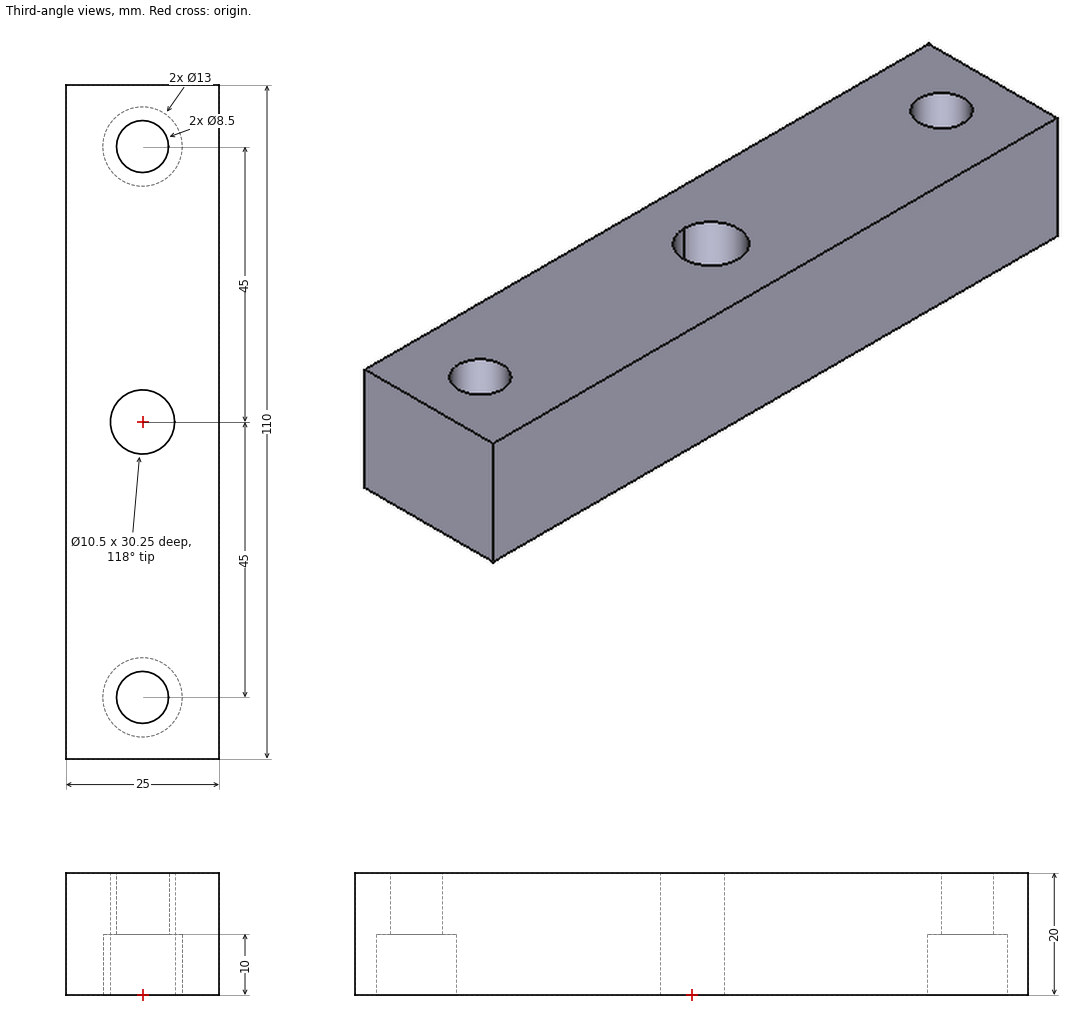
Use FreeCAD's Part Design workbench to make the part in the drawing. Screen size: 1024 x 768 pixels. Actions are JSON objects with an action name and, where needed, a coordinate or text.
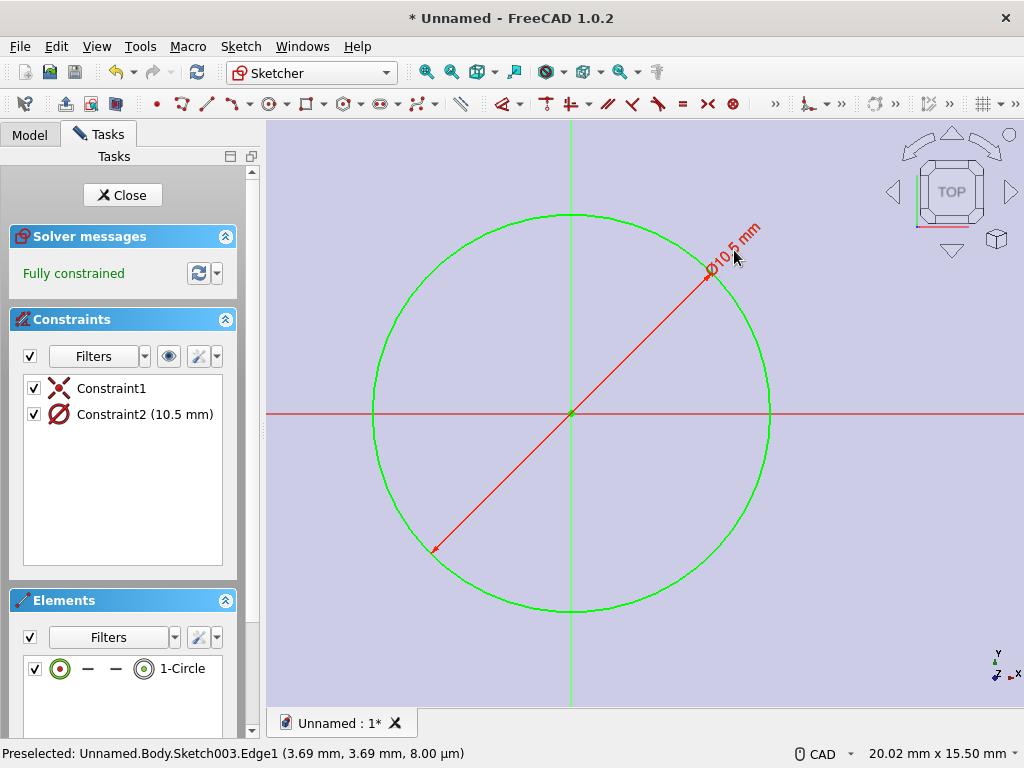
{"action": "left_click", "coordinate": [123, 195]}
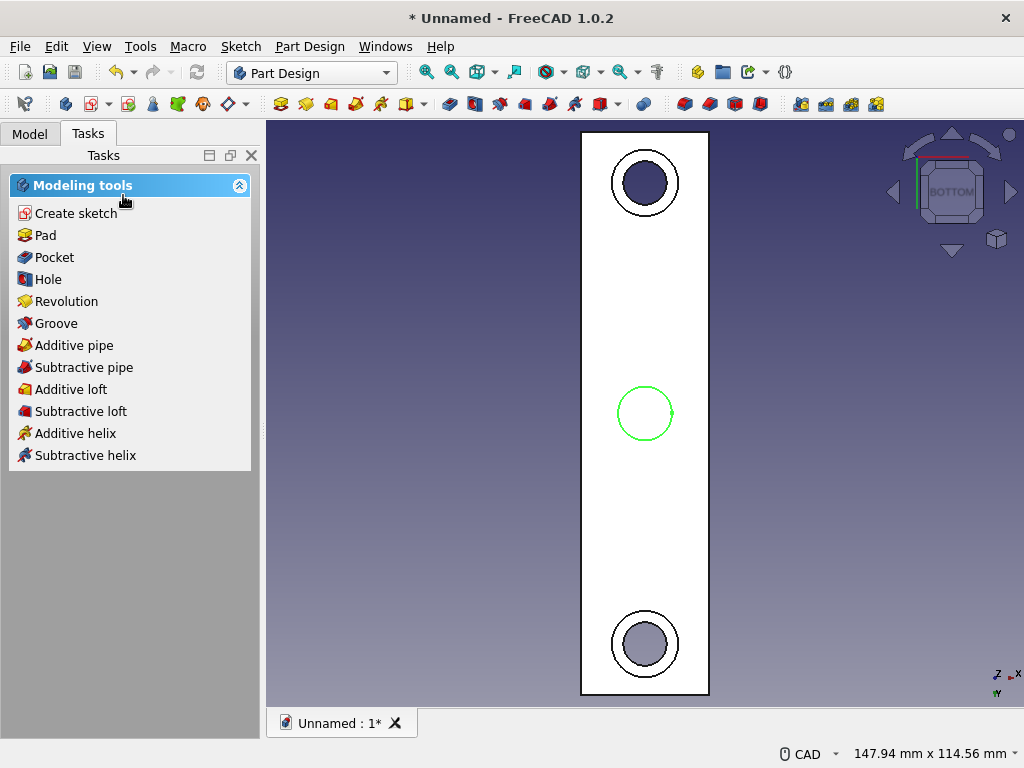
{"action": "left_click", "coordinate": [475, 104]}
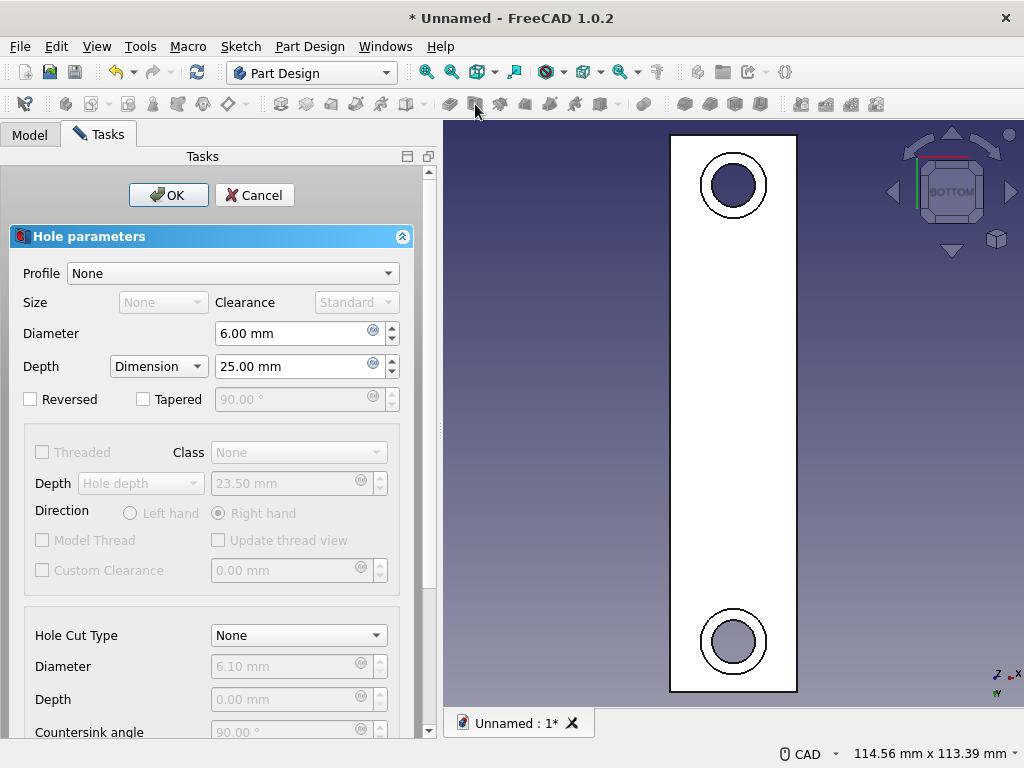
{"action": "triple_click", "coordinate": [300, 334]}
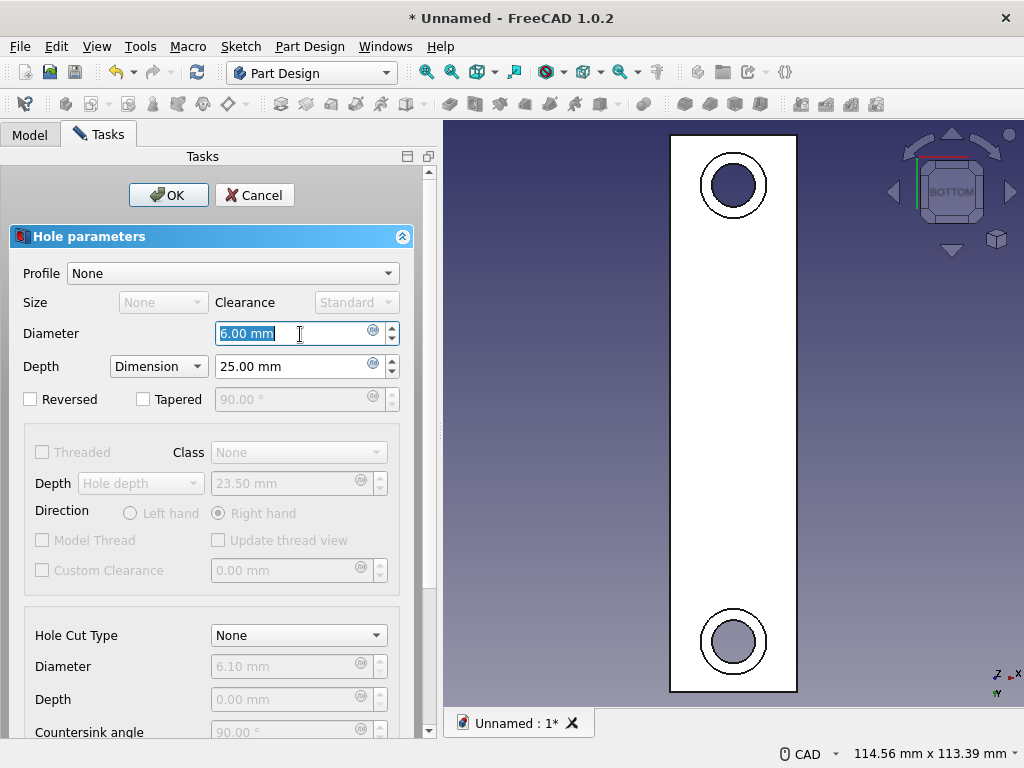
{"action": "type", "text": "10.5"}
{"action": "key", "text": "Tab"}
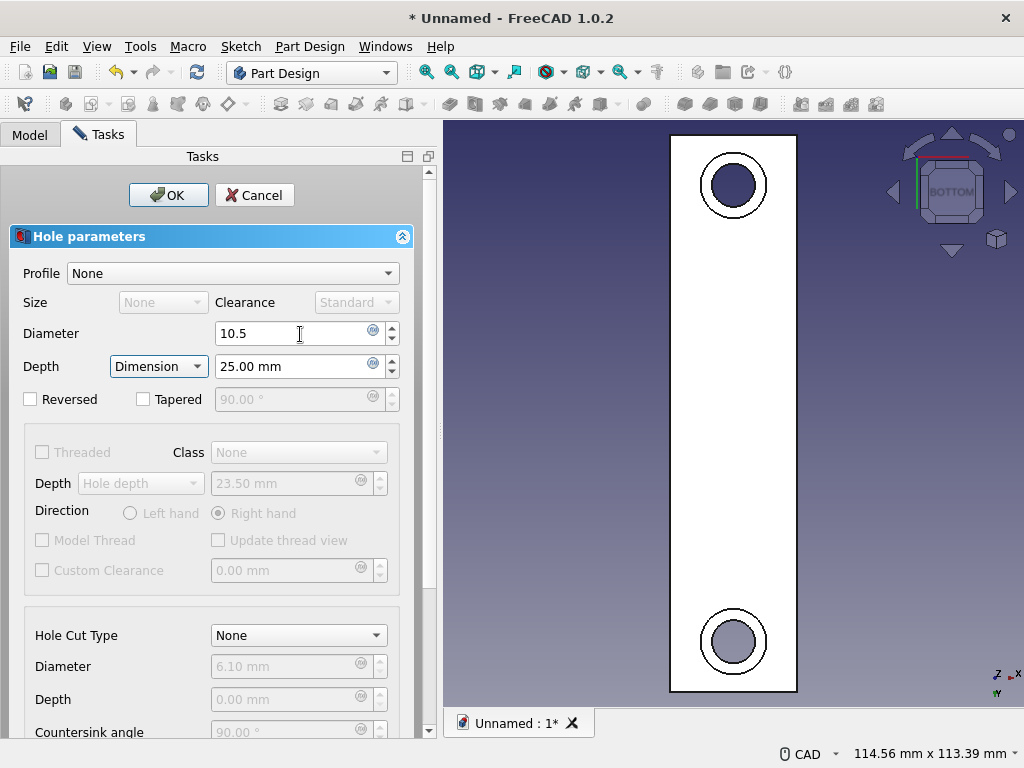
{"action": "triple_click", "coordinate": [300, 366]}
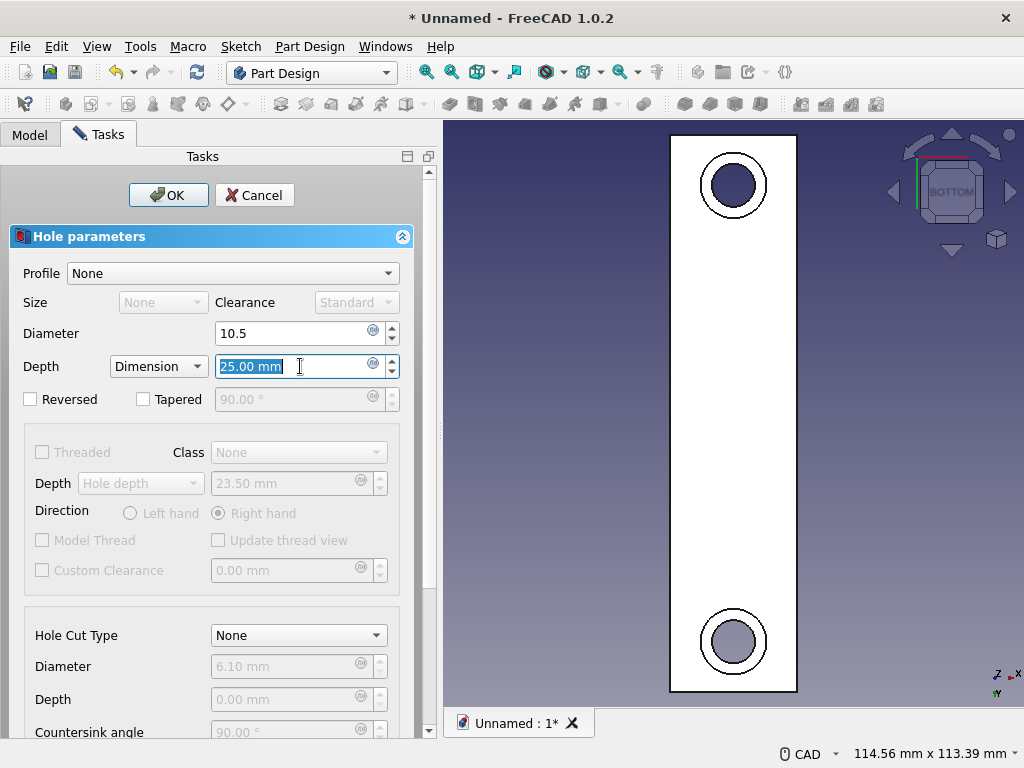
{"action": "type", "text": "30.25"}
{"action": "key", "text": "Tab"}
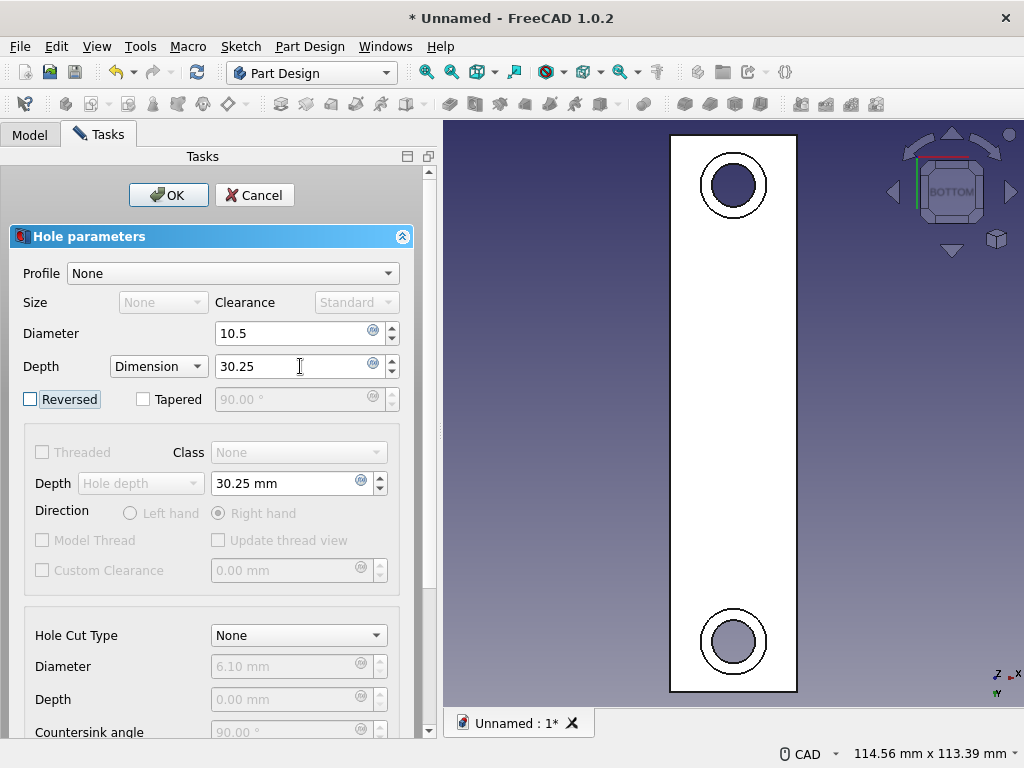
{"action": "left_click", "coordinate": [31, 399]}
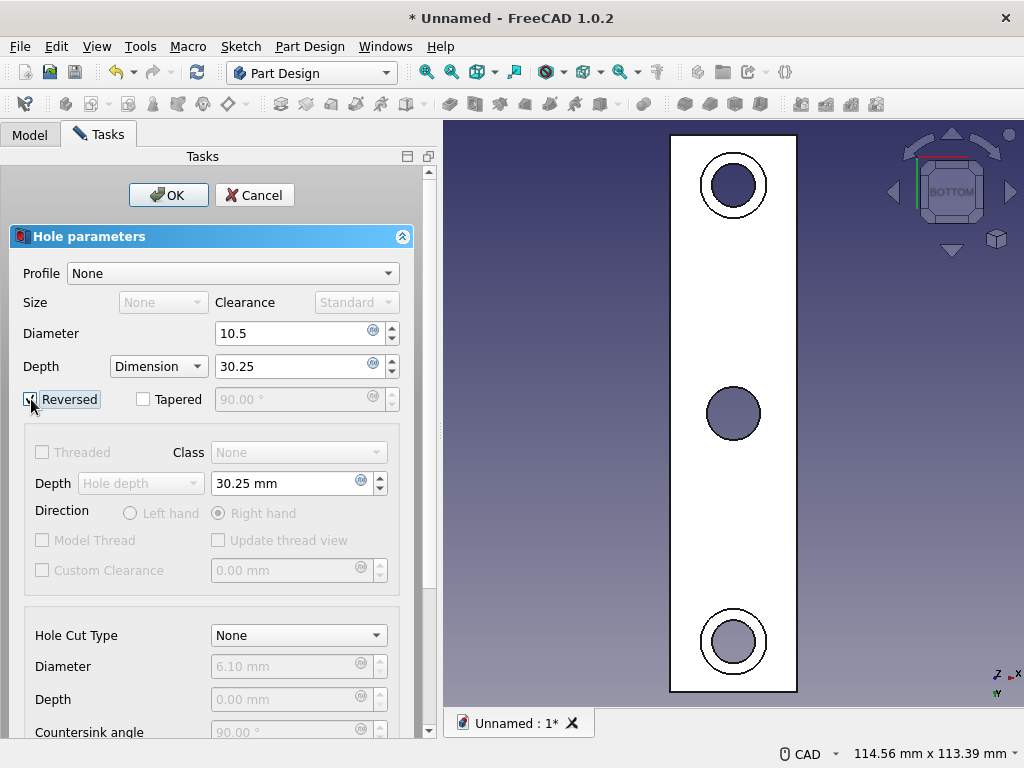
{"action": "left_click", "coordinate": [169, 195]}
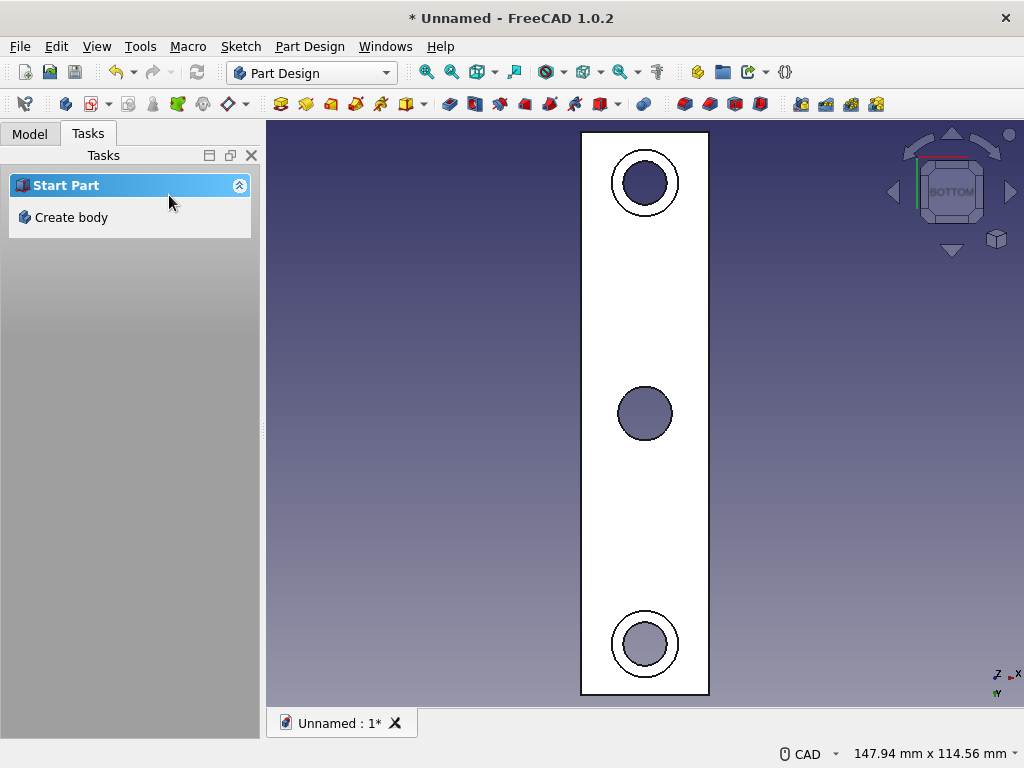
{"action": "key", "text": "0"}